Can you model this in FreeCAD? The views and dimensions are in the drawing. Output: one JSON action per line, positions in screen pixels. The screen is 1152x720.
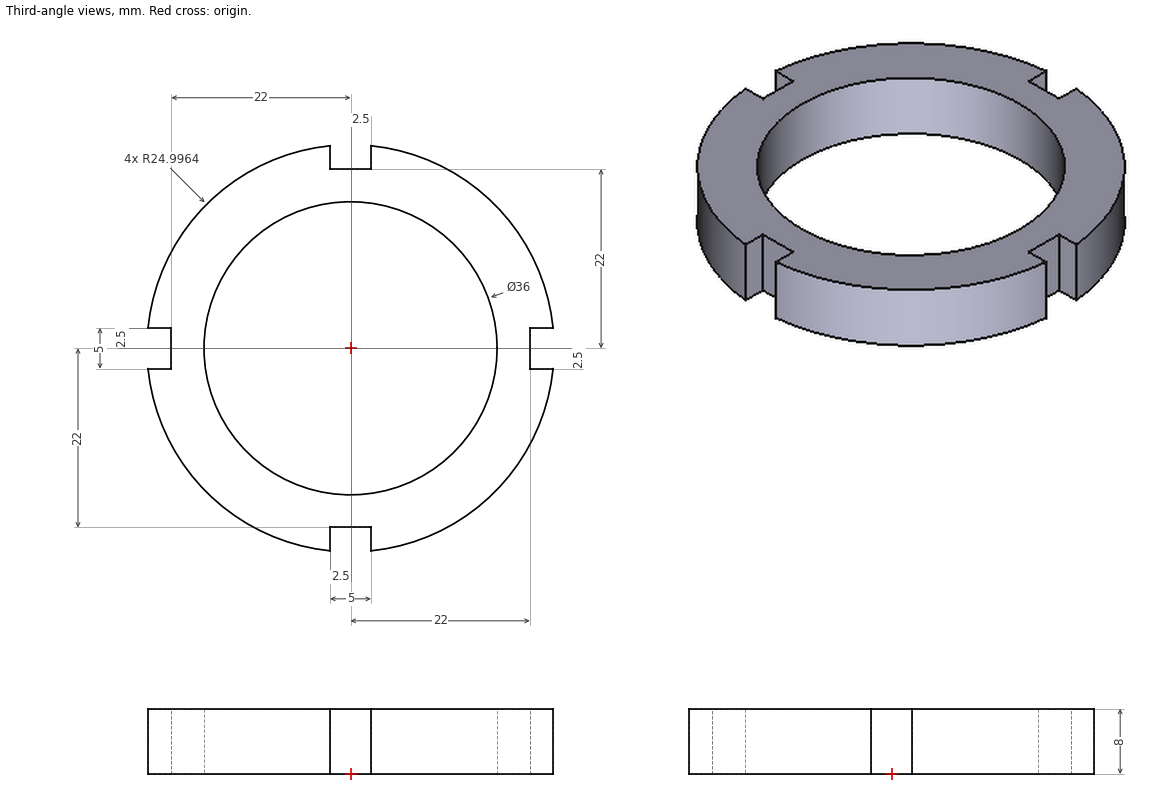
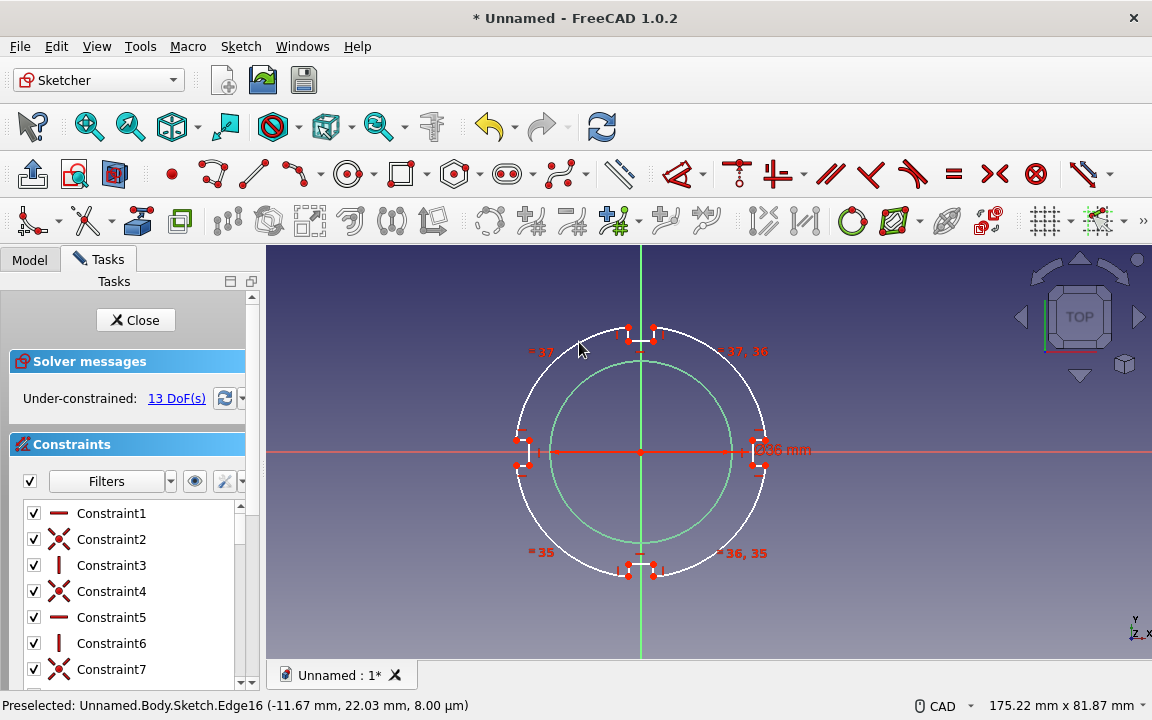
{"action": "key", "text": "d"}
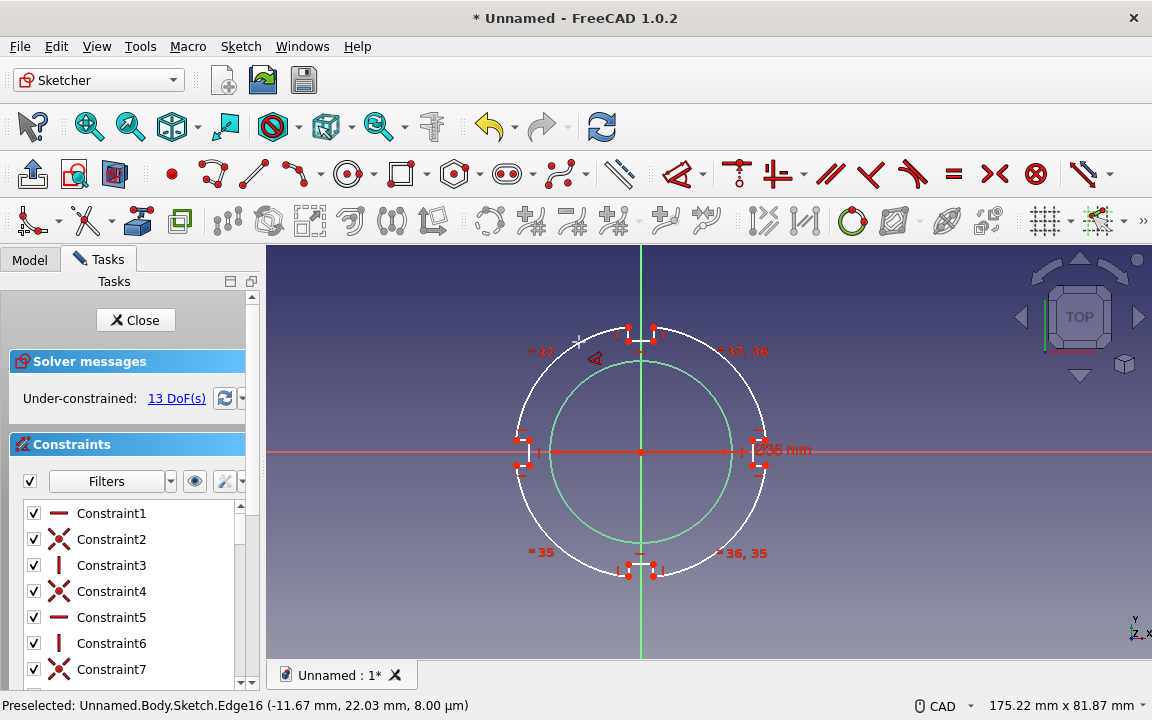
{"action": "left_click", "coordinate": [532, 514]}
{"action": "left_click", "coordinate": [504, 530]}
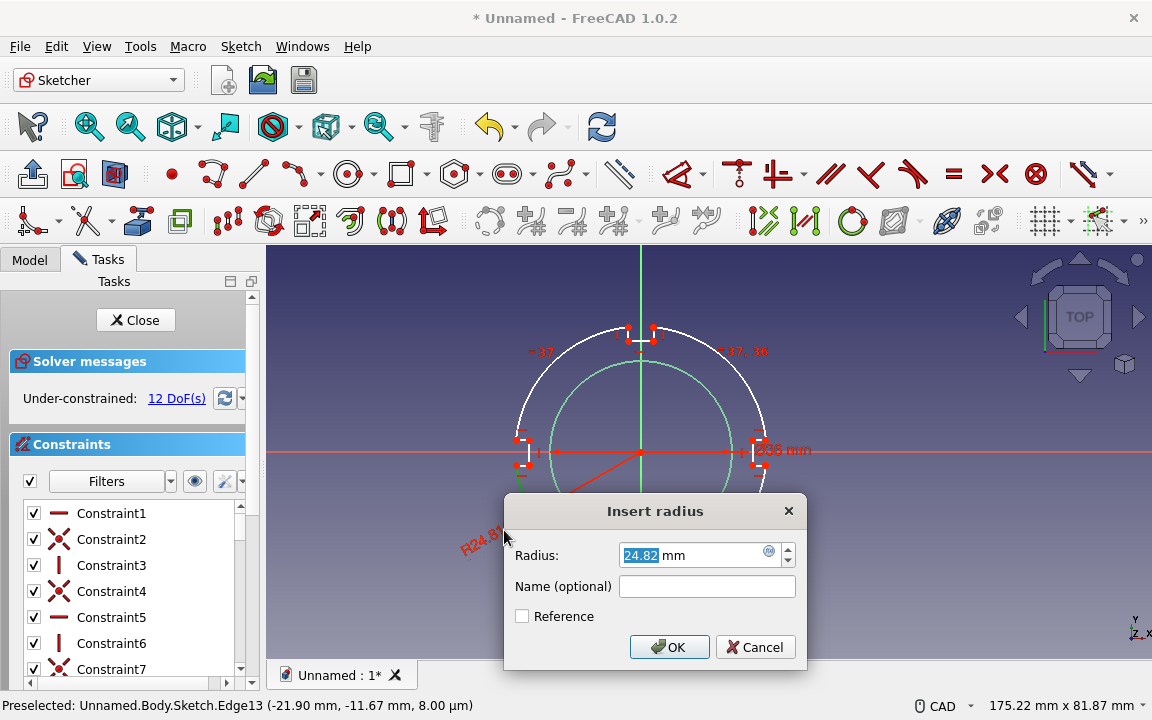
{"action": "type", "text": "24.9964"}
{"action": "key", "text": "Return"}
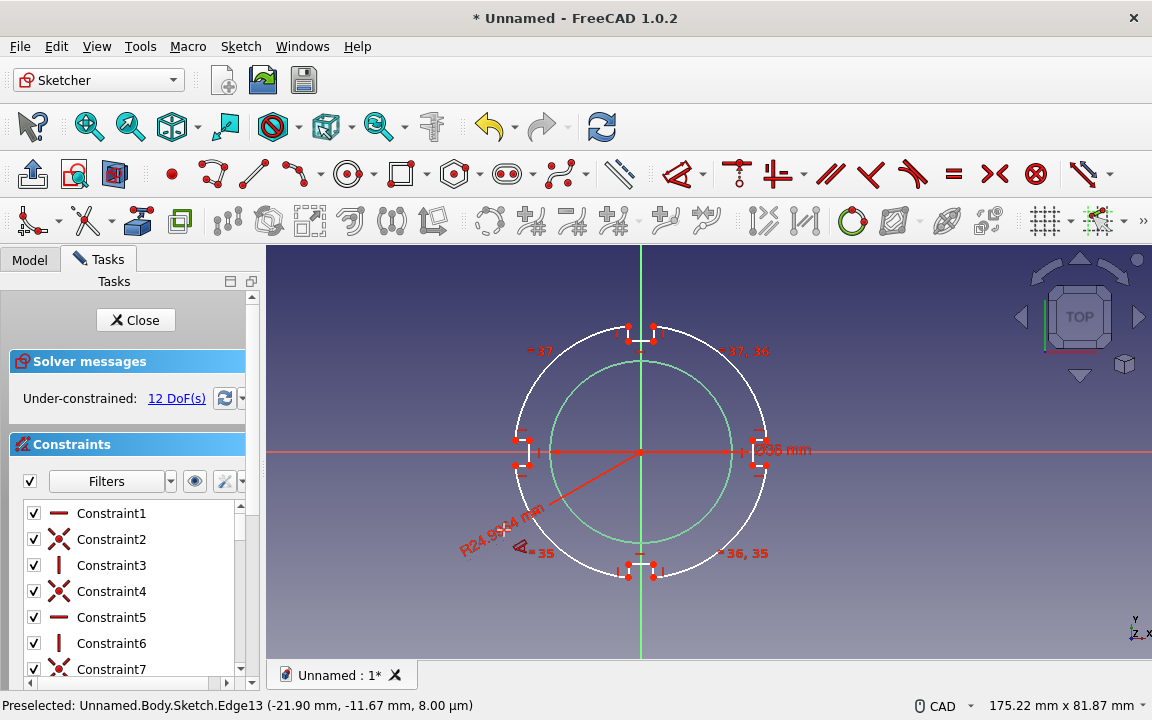
{"action": "scroll", "coordinate": [529, 450], "scroll_direction": "up", "scroll_amount": 3}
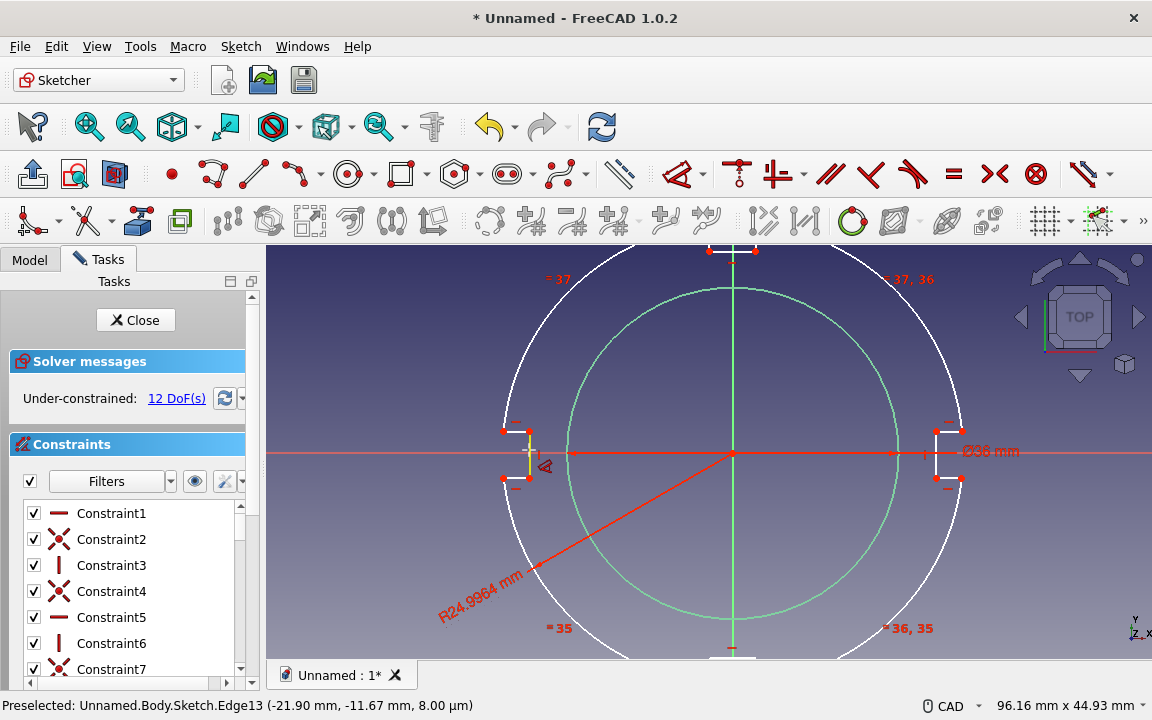
{"action": "left_click", "coordinate": [530, 450]}
{"action": "left_click", "coordinate": [472, 439]}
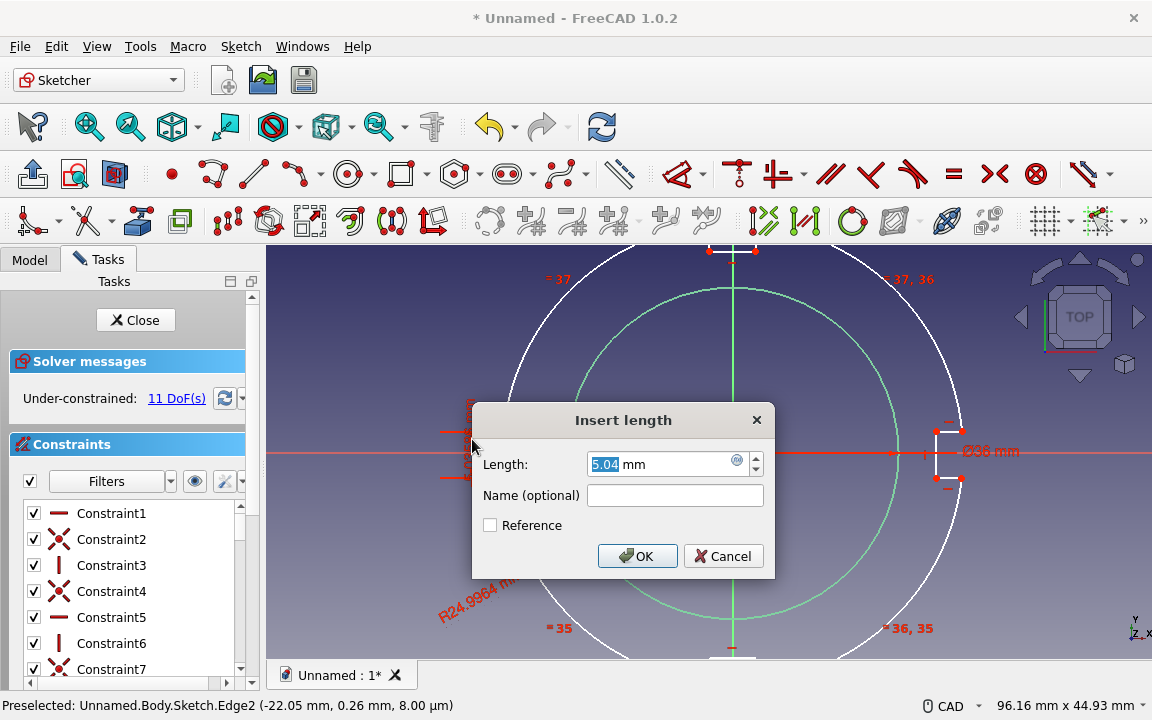
{"action": "type", "text": "5"}
{"action": "key", "text": "Return"}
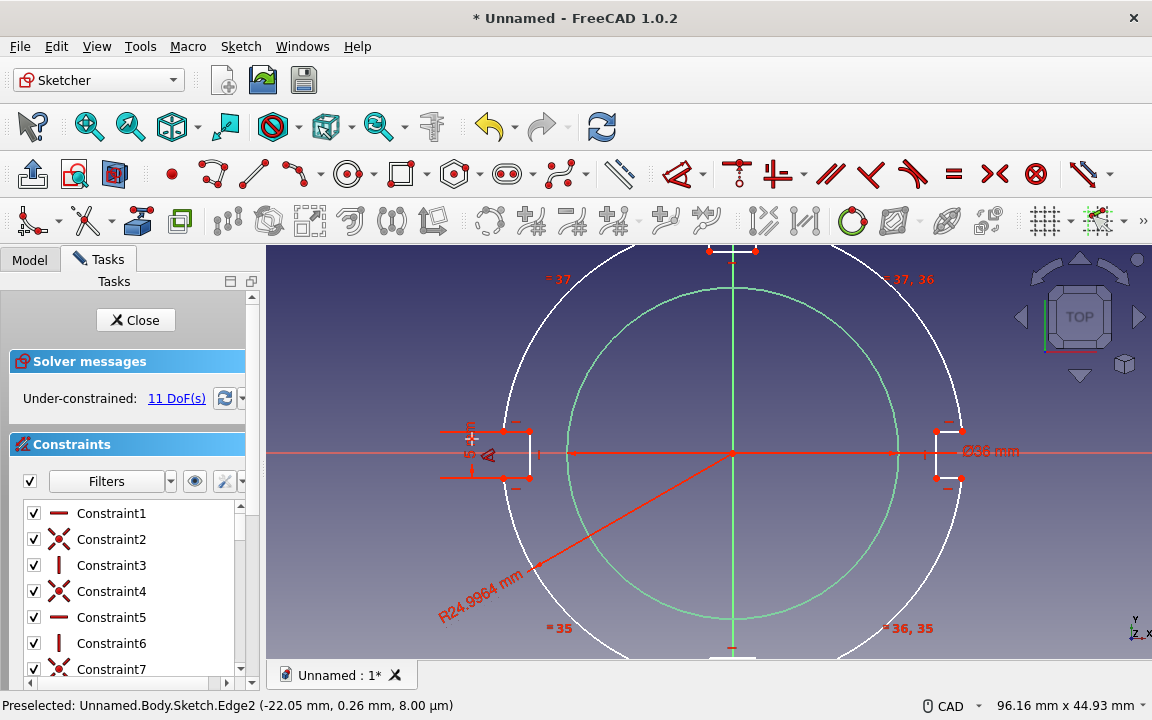
{"action": "scroll", "coordinate": [528, 450], "scroll_direction": "down", "scroll_amount": 3}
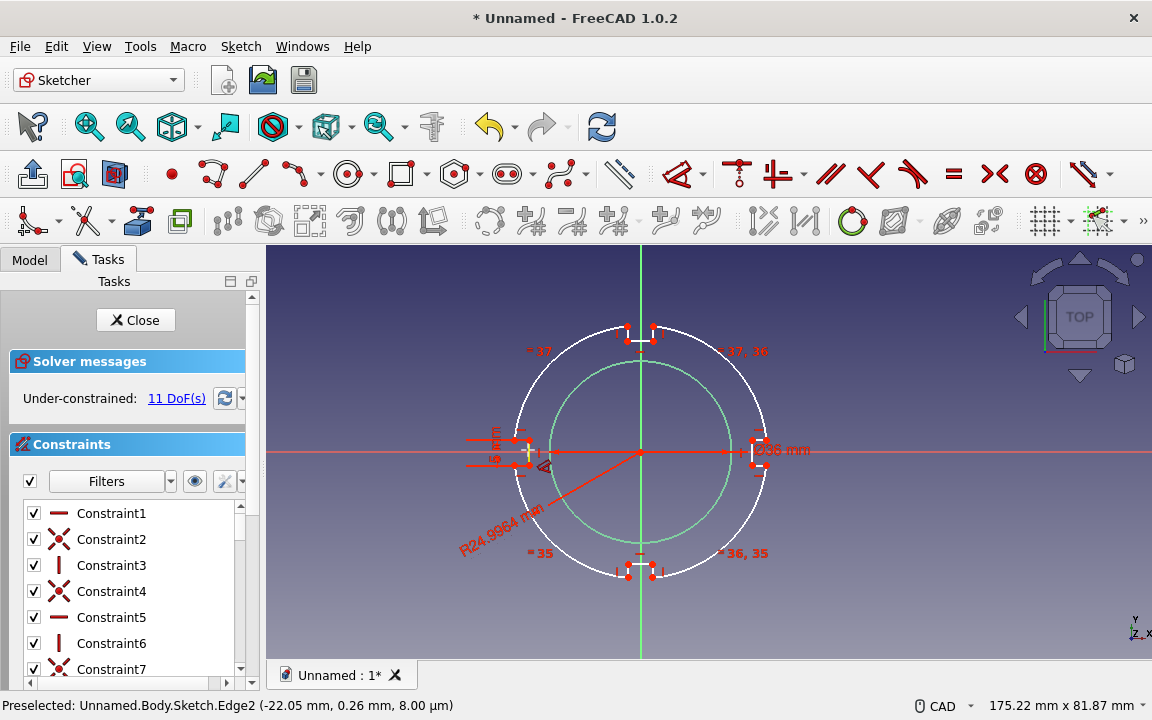
{"action": "scroll", "coordinate": [635, 564], "scroll_direction": "up", "scroll_amount": 6}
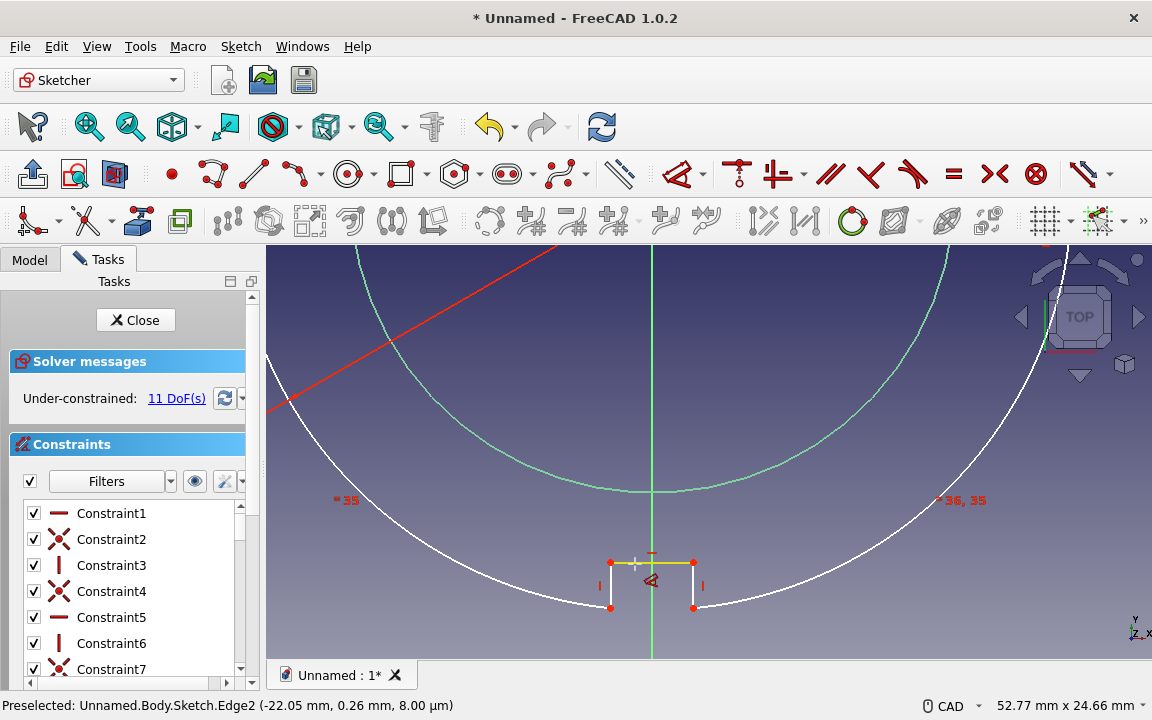
{"action": "left_click", "coordinate": [636, 563]}
{"action": "left_click", "coordinate": [633, 597]}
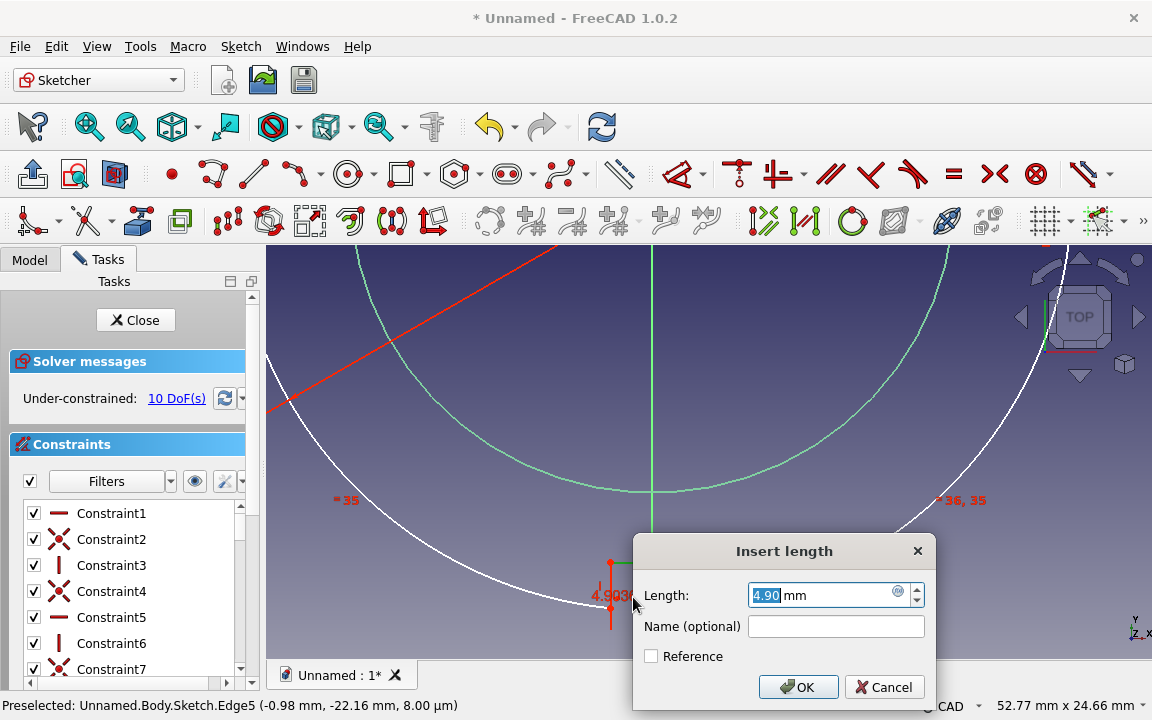
{"action": "type", "text": "5"}
{"action": "key", "text": "Return"}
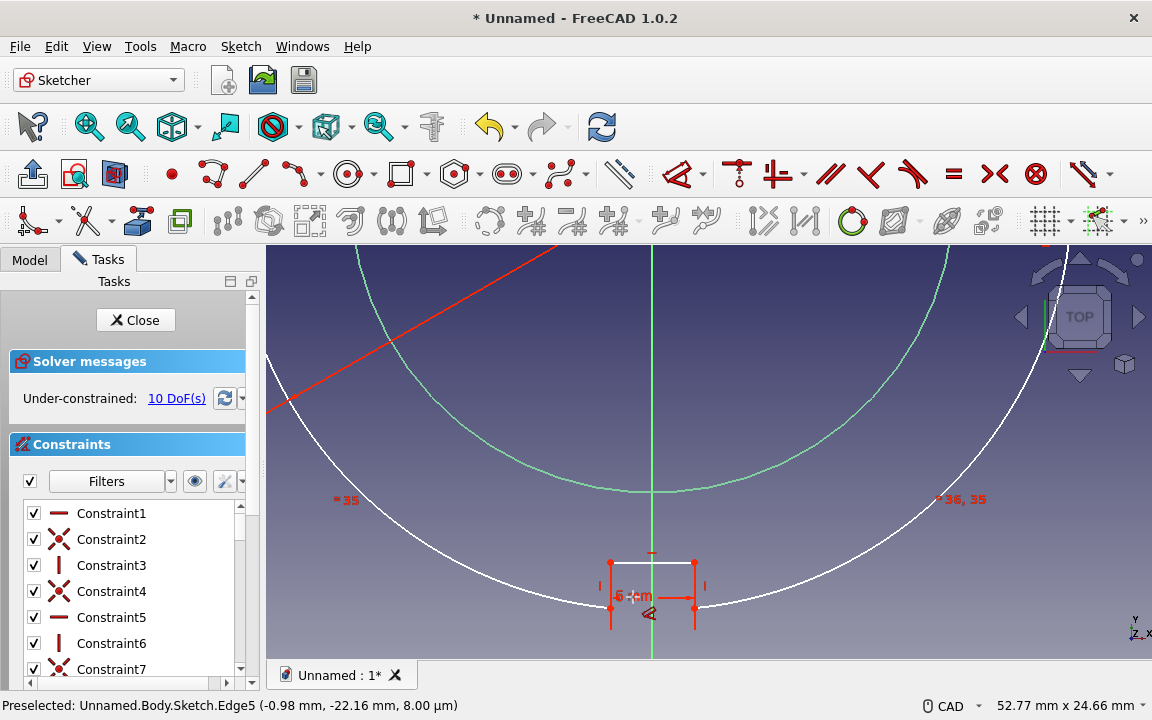
{"action": "scroll", "coordinate": [635, 565], "scroll_direction": "down", "scroll_amount": 6}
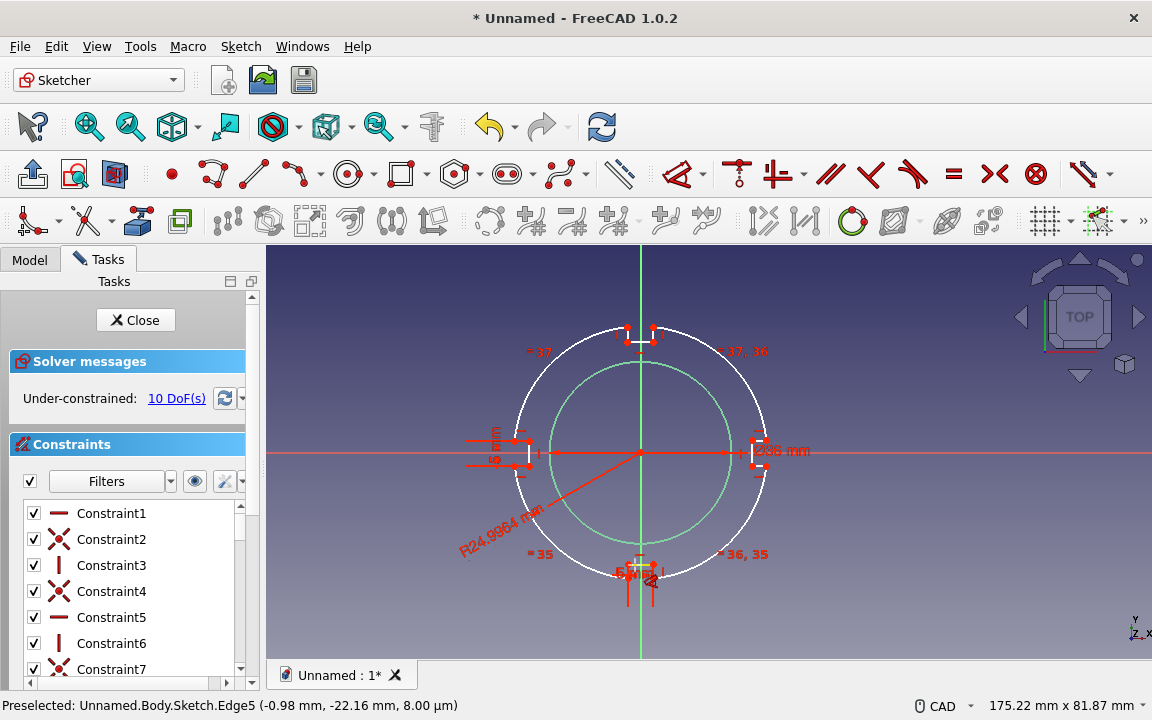
{"action": "scroll", "coordinate": [752, 459], "scroll_direction": "up", "scroll_amount": 5}